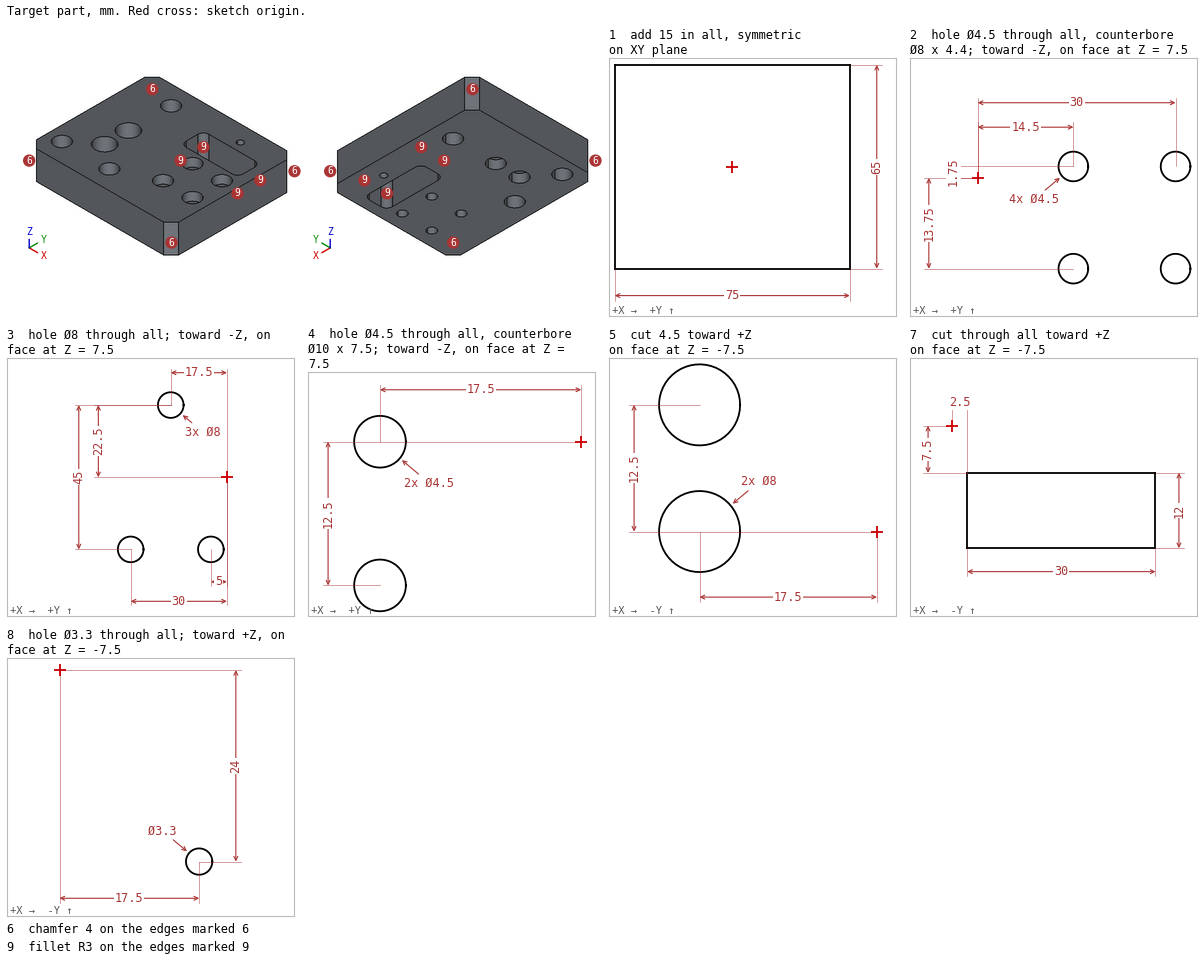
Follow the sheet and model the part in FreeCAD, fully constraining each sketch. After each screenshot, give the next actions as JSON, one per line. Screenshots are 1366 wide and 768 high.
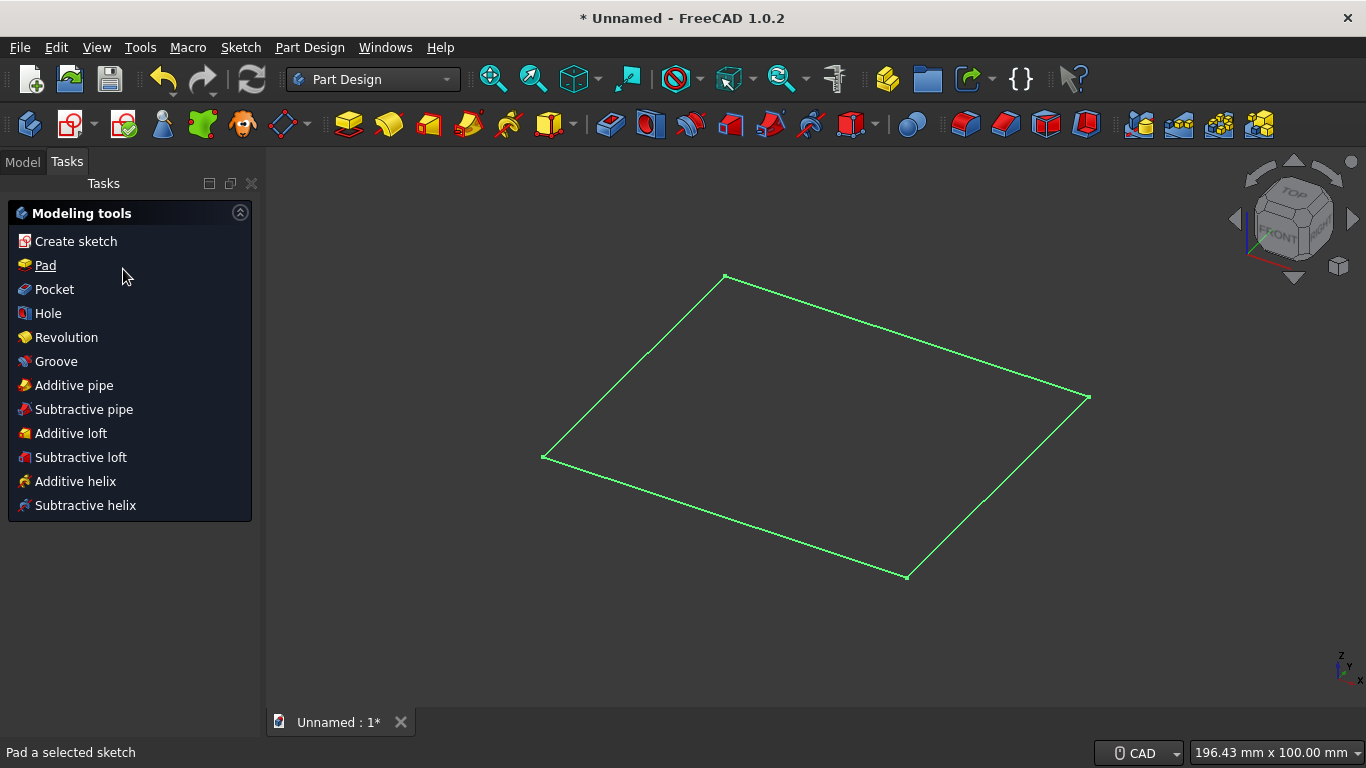
{"action": "left_click", "coordinate": [350, 124]}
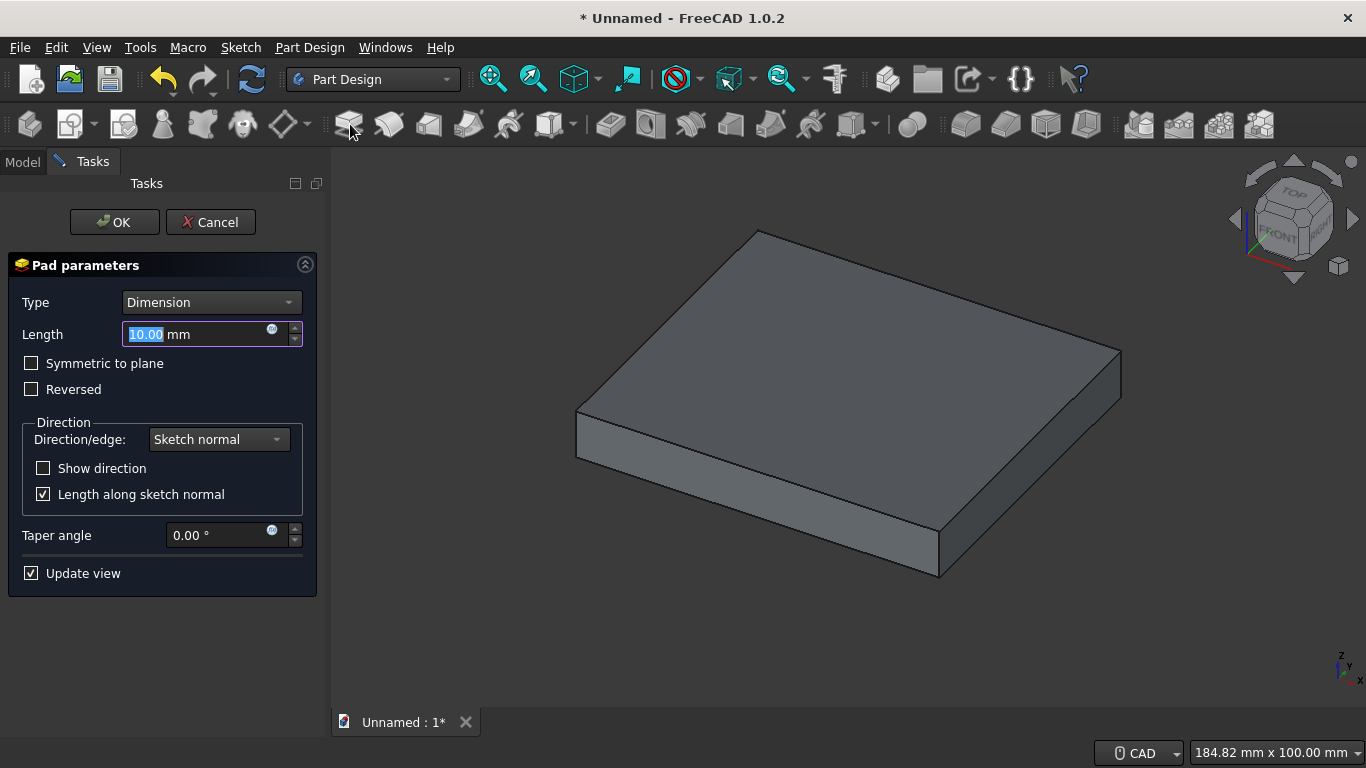
{"action": "type", "text": "15"}
{"action": "key", "text": "Tab"}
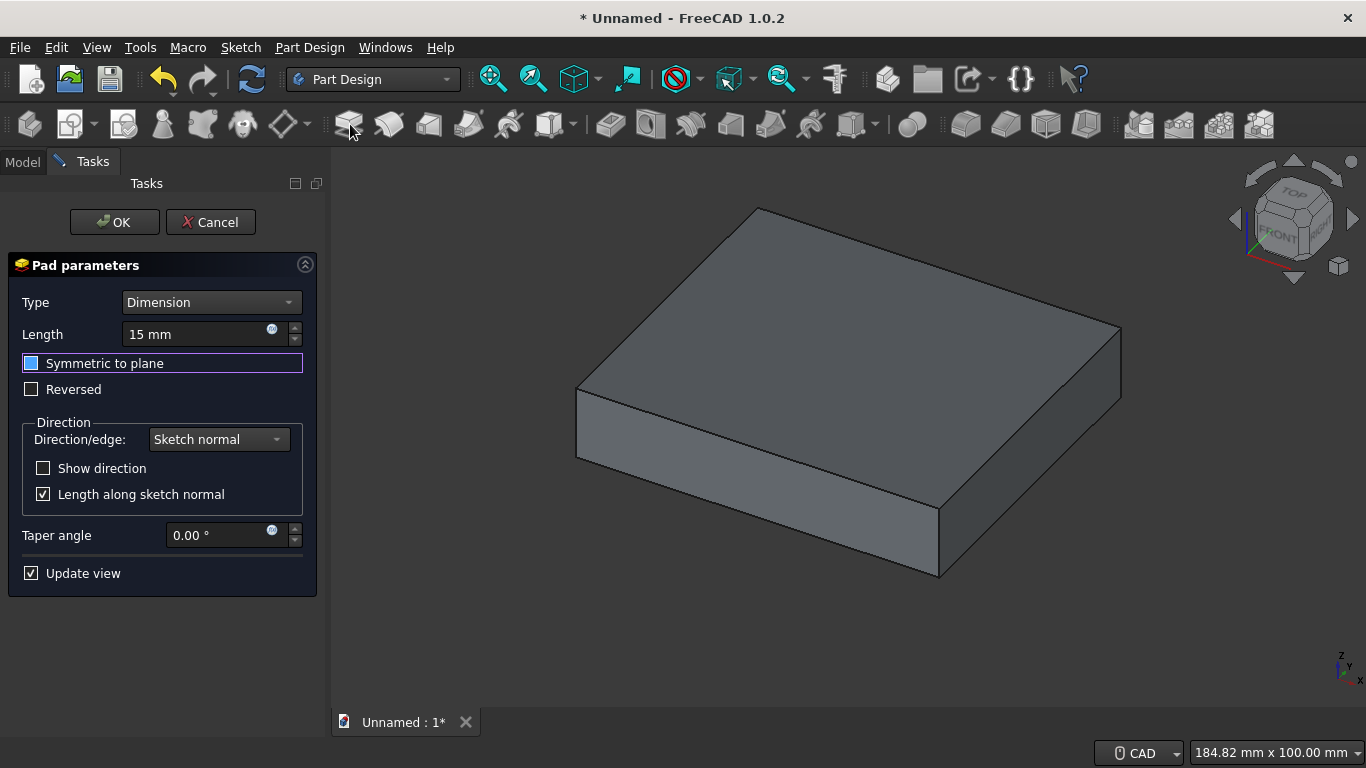
{"action": "left_click", "coordinate": [30, 363]}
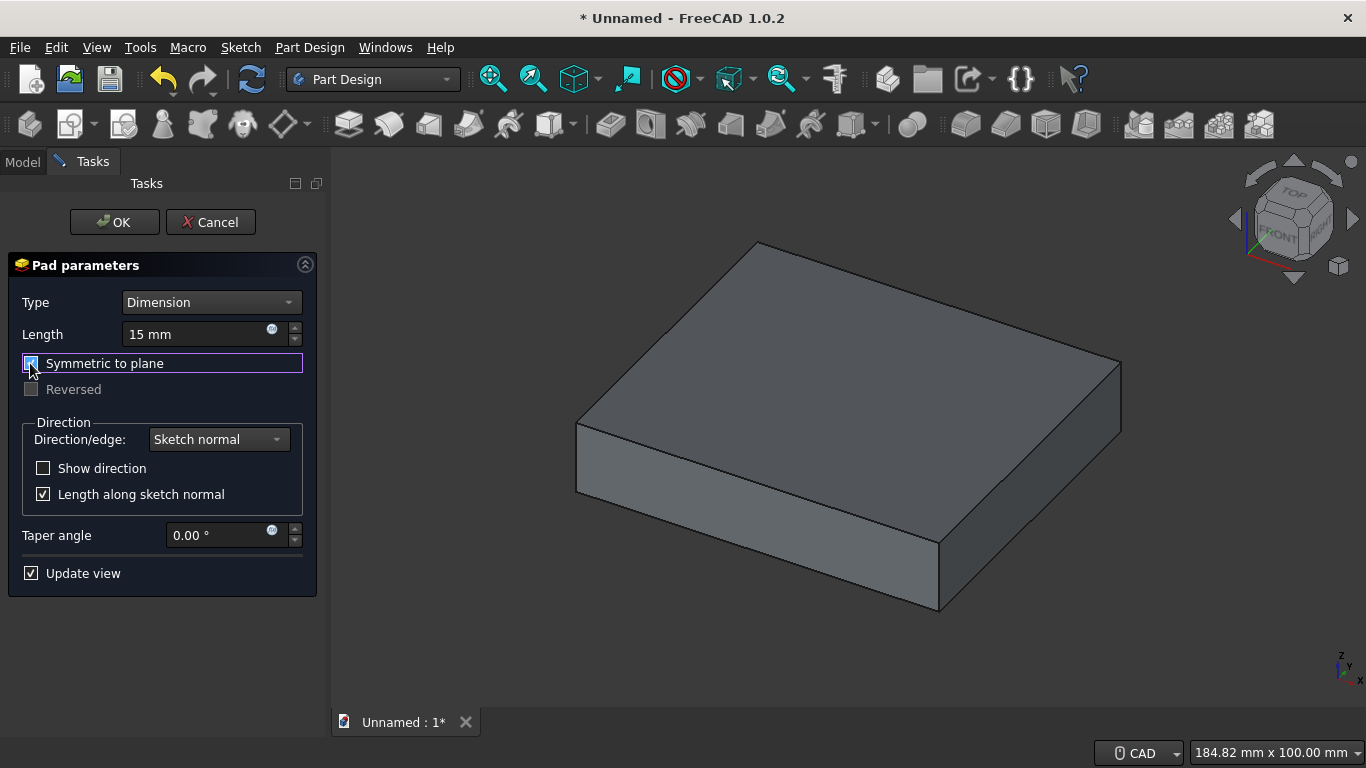
{"action": "left_click", "coordinate": [115, 222]}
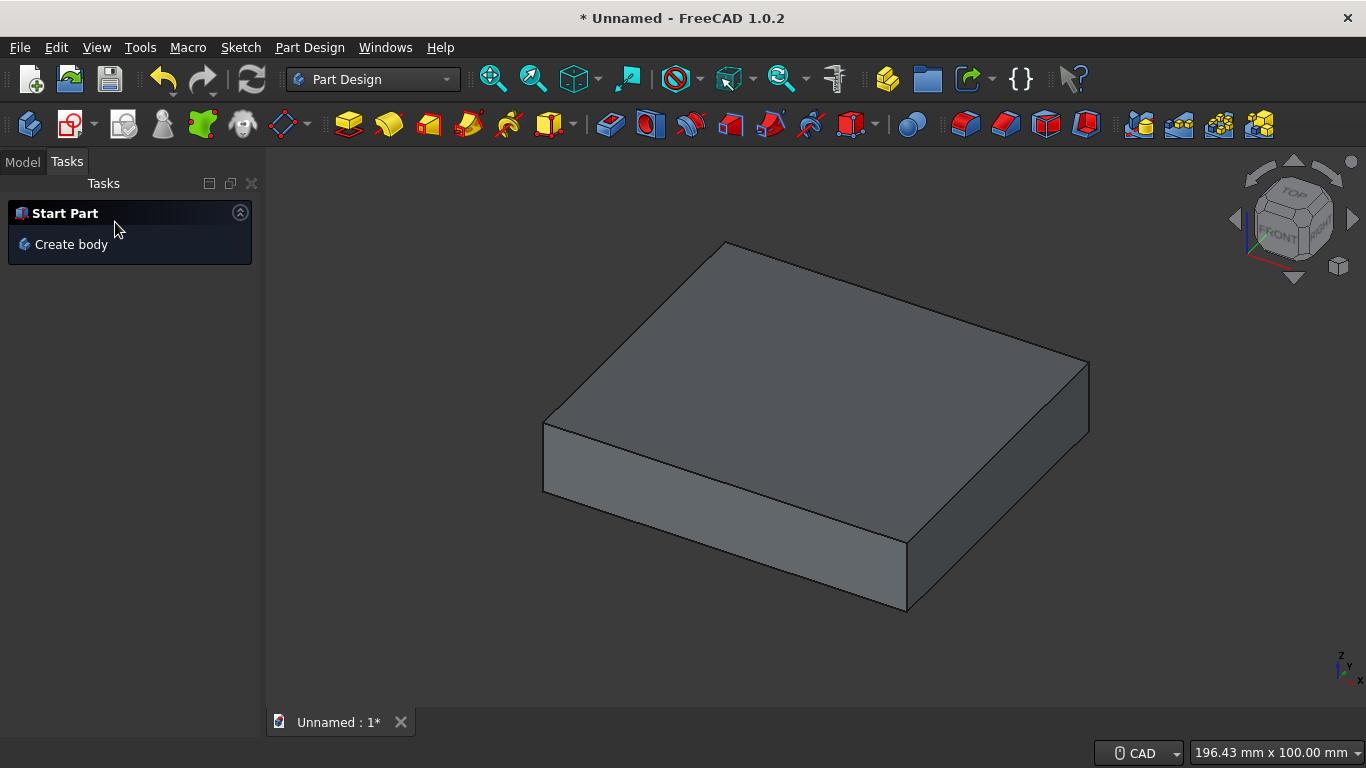
{"action": "left_click", "coordinate": [816, 392]}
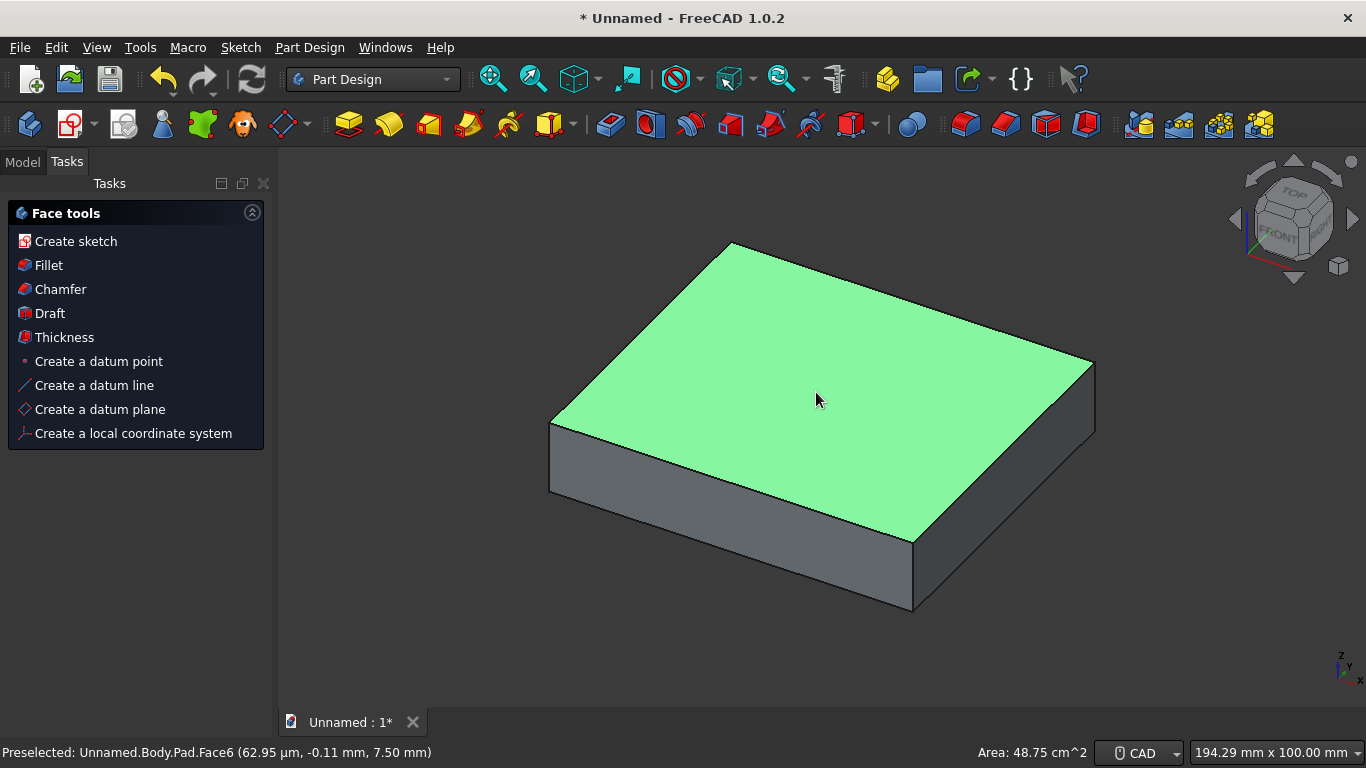
{"action": "left_click", "coordinate": [70, 124]}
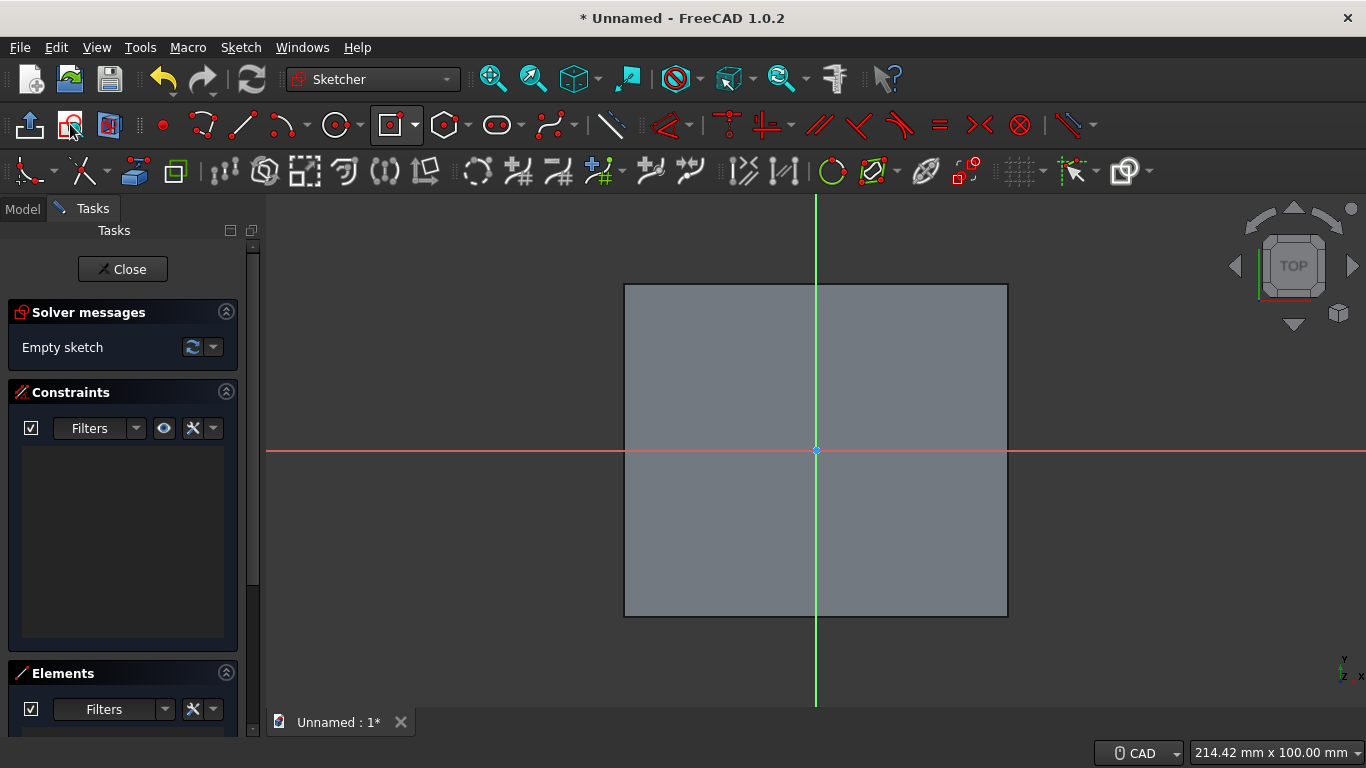
{"action": "scroll", "coordinate": [964, 495], "scroll_direction": "up", "scroll_amount": 6}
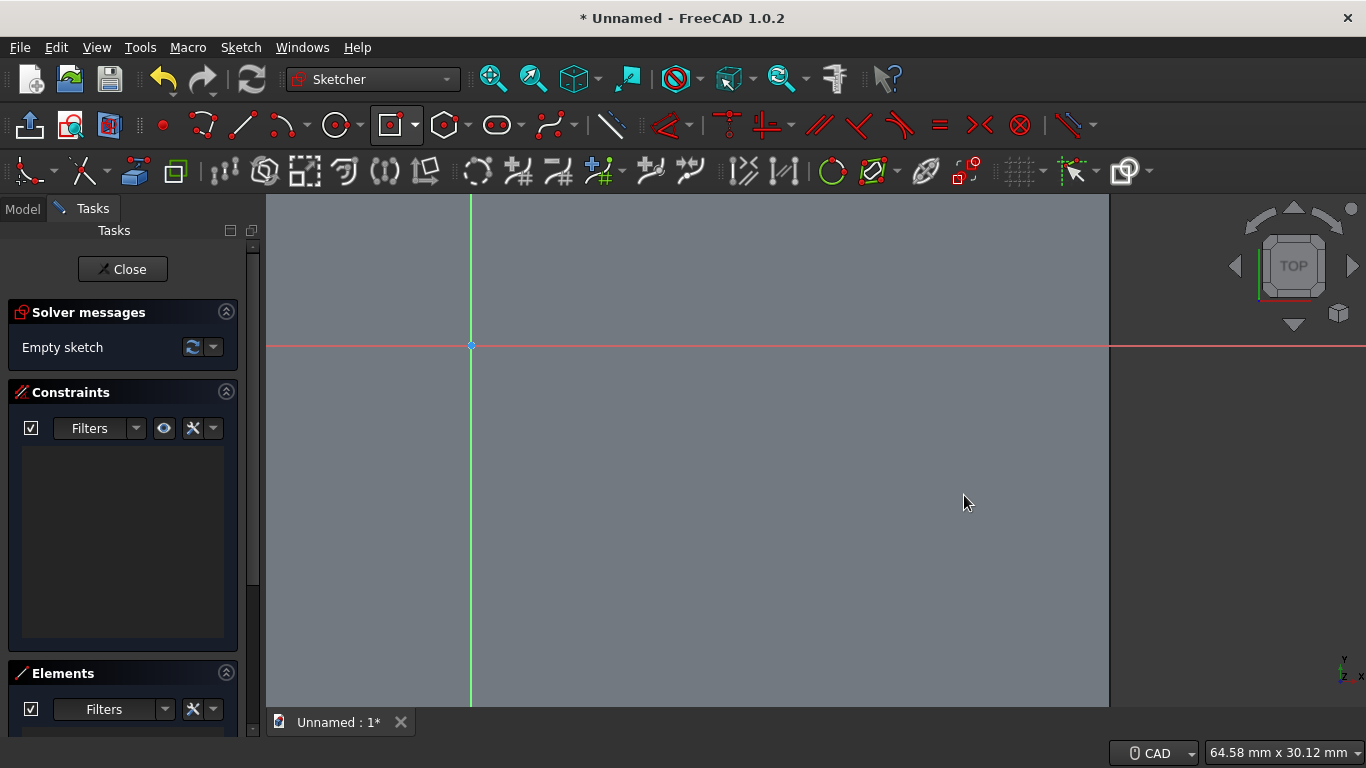
{"action": "left_click", "coordinate": [336, 126]}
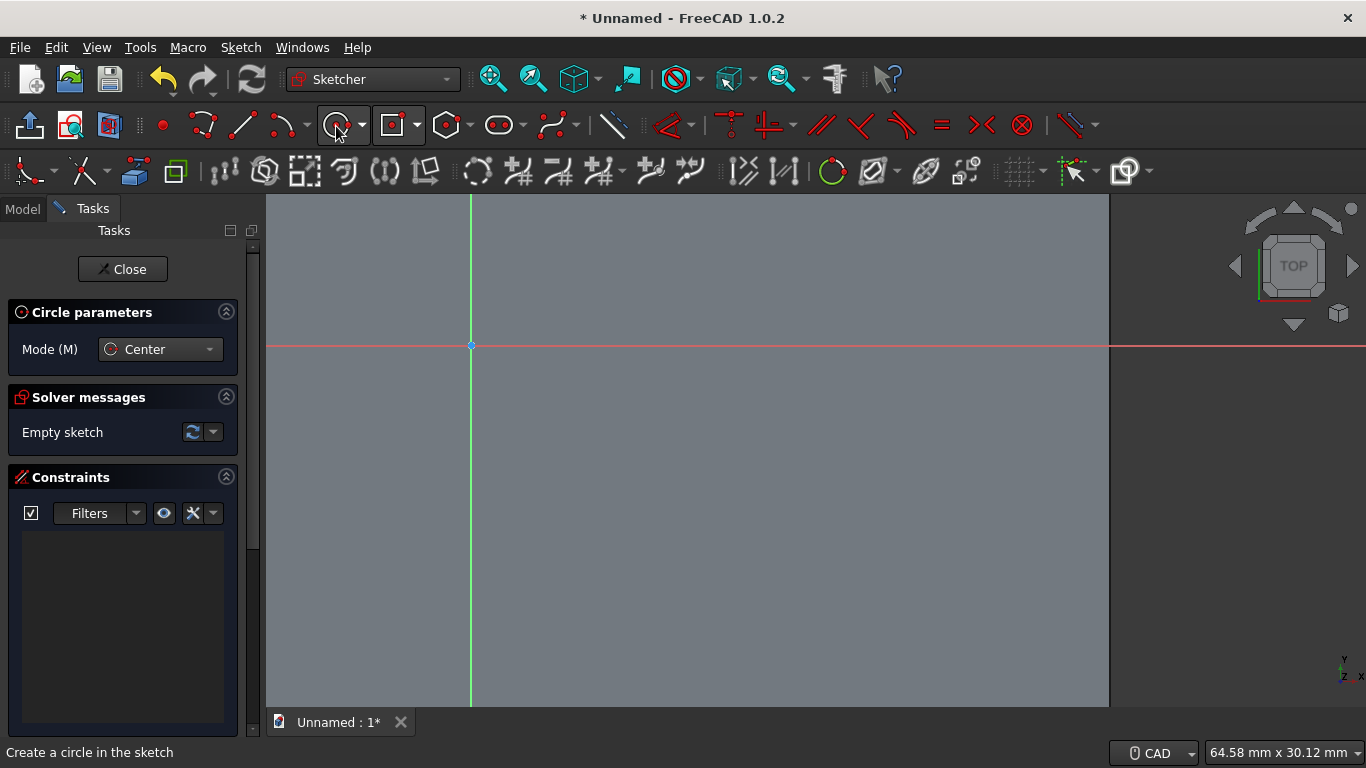
{"action": "left_click", "coordinate": [718, 316]}
{"action": "mouse_move", "coordinate": [745, 289]}